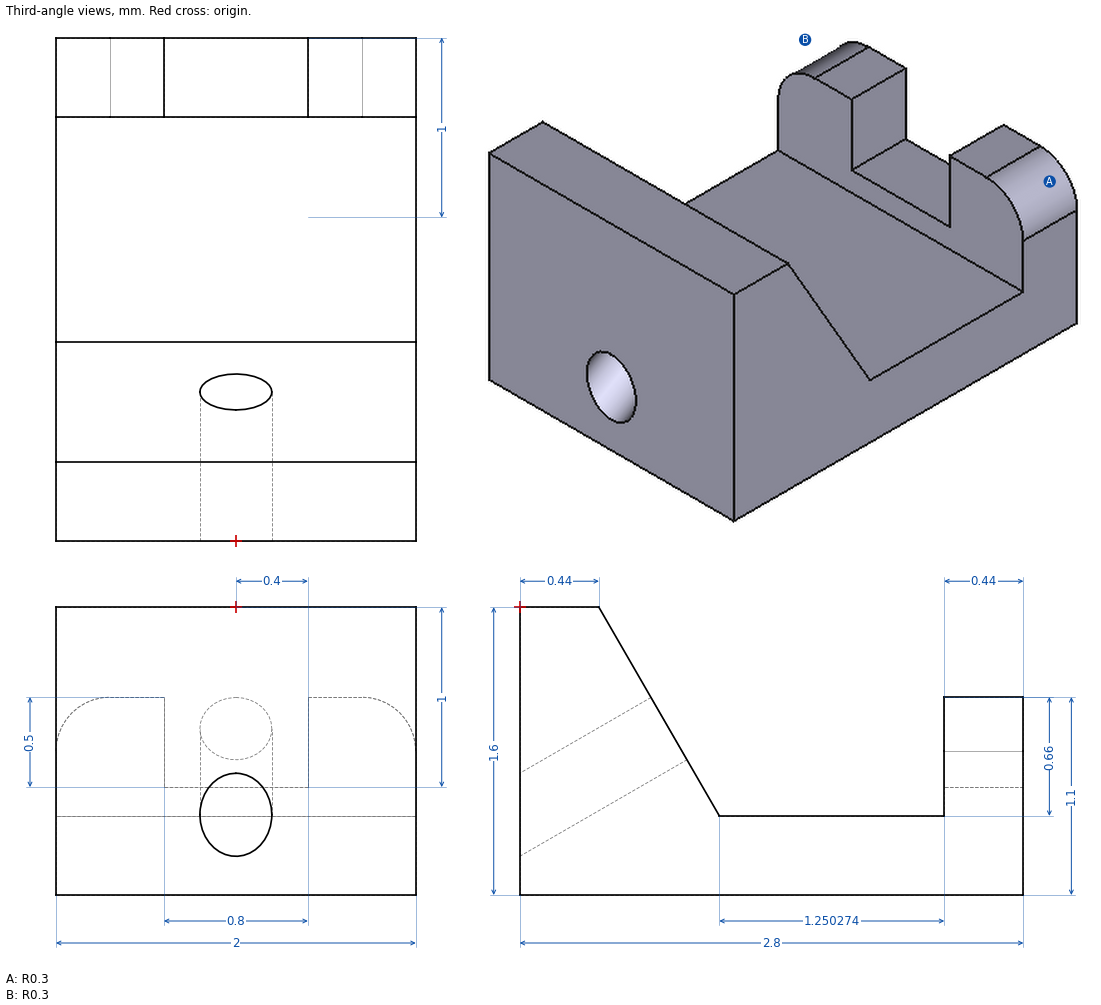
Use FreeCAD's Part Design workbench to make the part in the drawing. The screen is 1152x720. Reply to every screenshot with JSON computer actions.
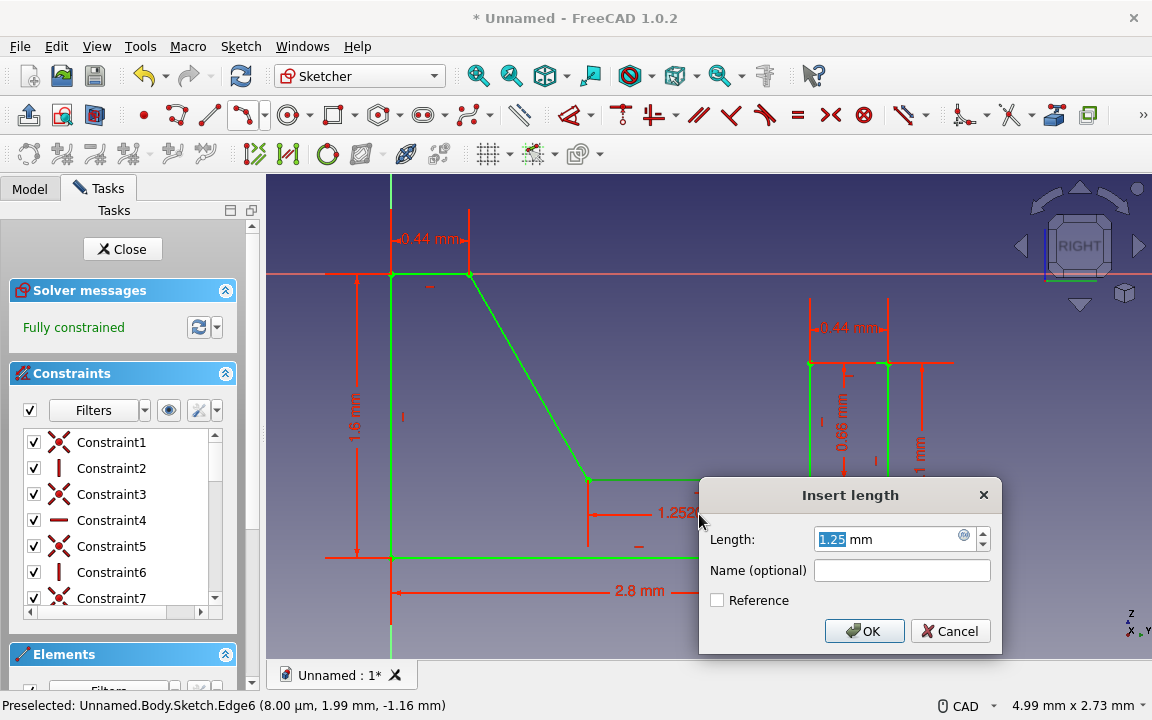
{"action": "type", "text": "1.250274"}
{"action": "key", "text": "Return"}
{"action": "key", "text": "Escape"}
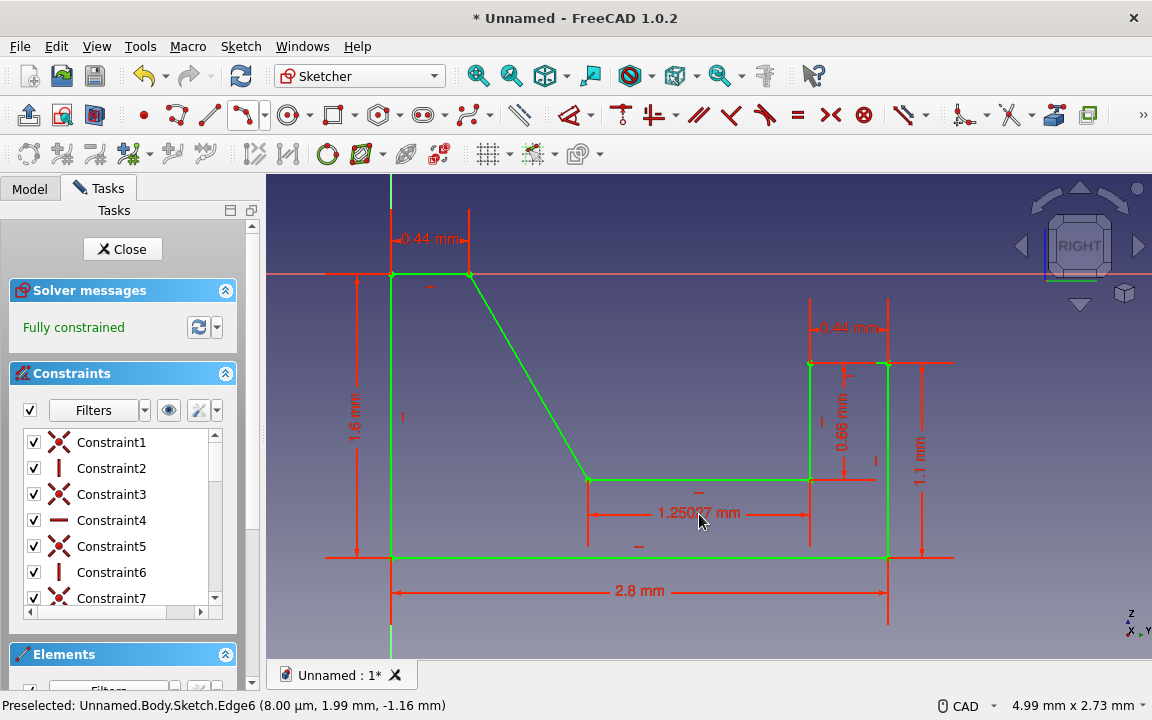
{"action": "left_click", "coordinate": [123, 249]}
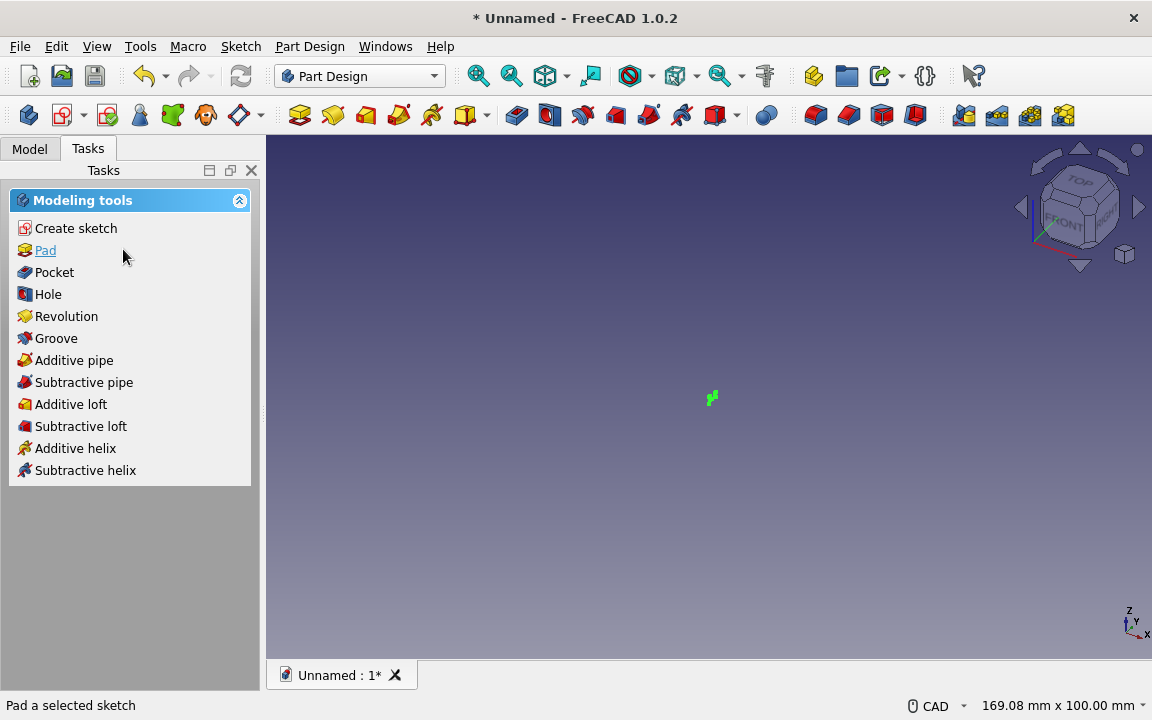
{"action": "left_click", "coordinate": [300, 116]}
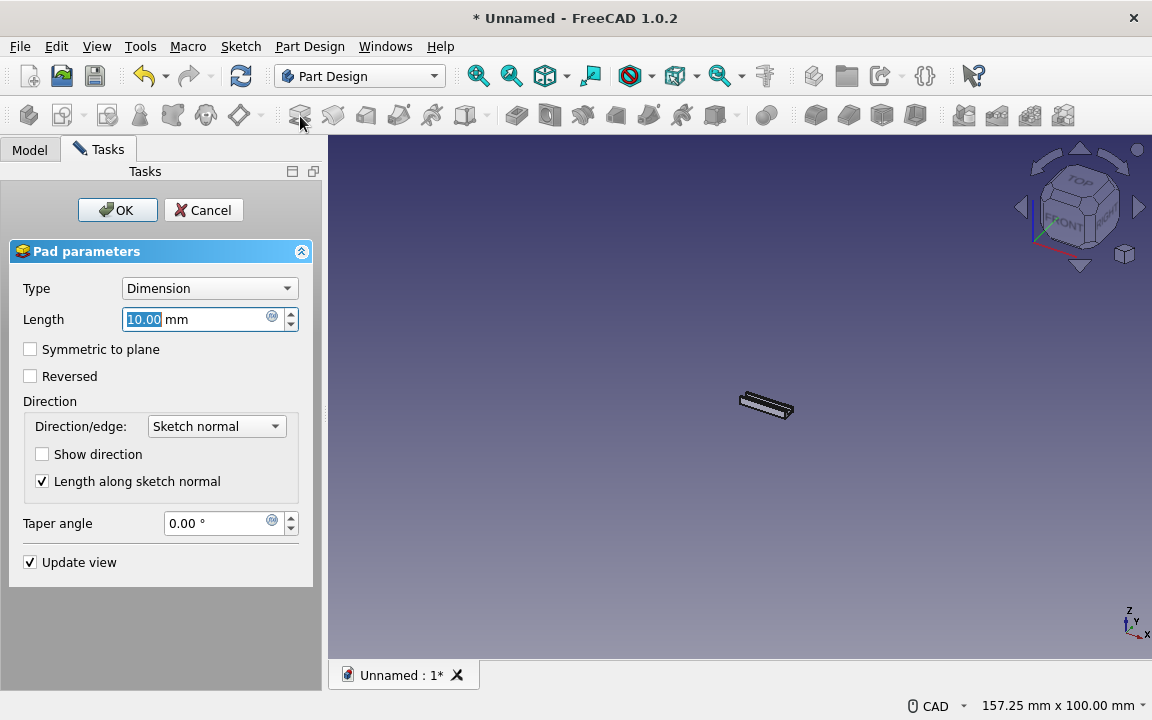
{"action": "type", "text": "2"}
{"action": "key", "text": "Tab"}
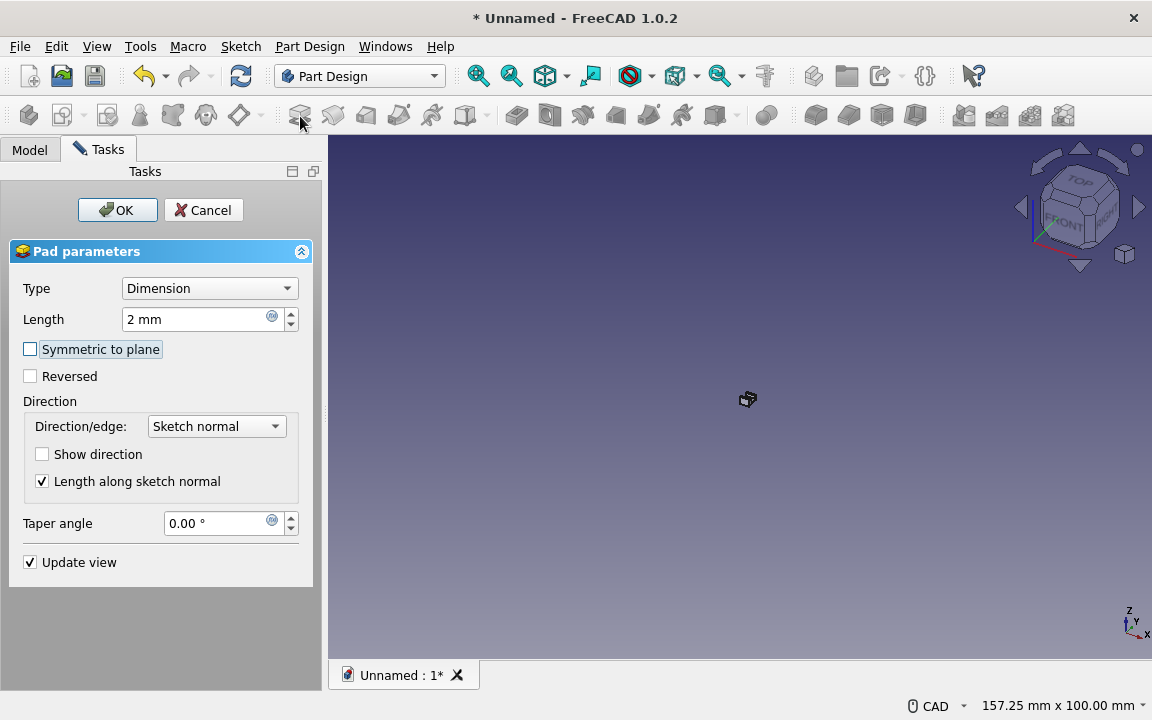
{"action": "left_click", "coordinate": [31, 349]}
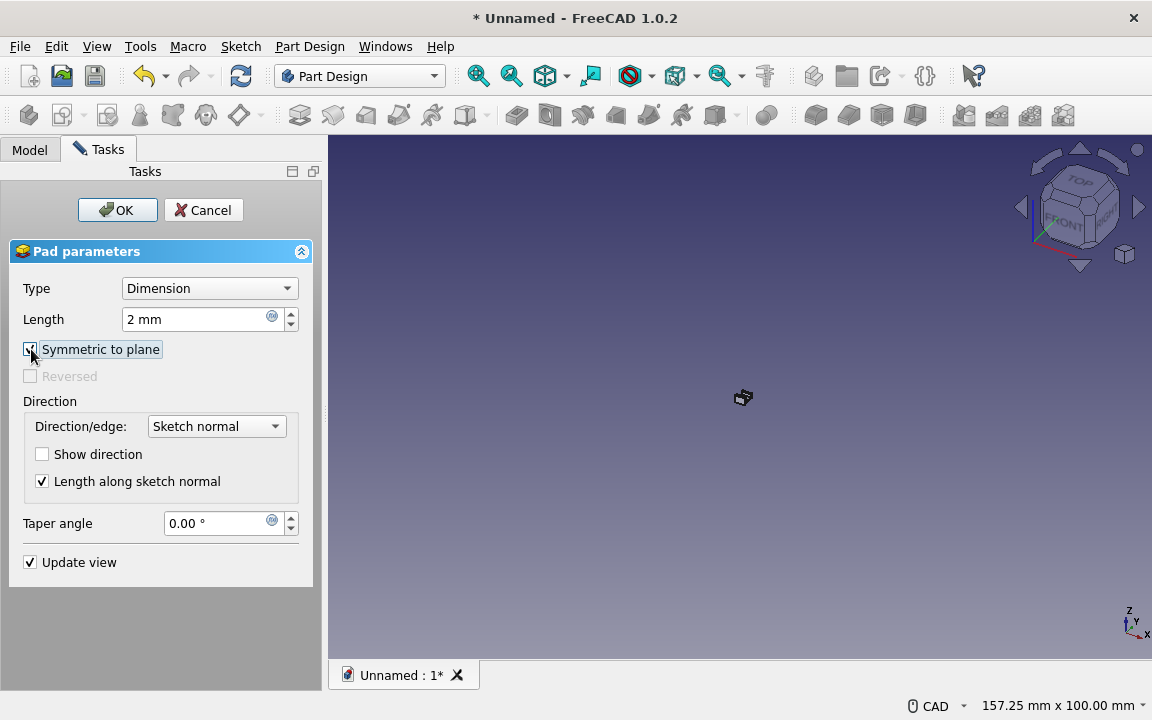
{"action": "left_click", "coordinate": [118, 210]}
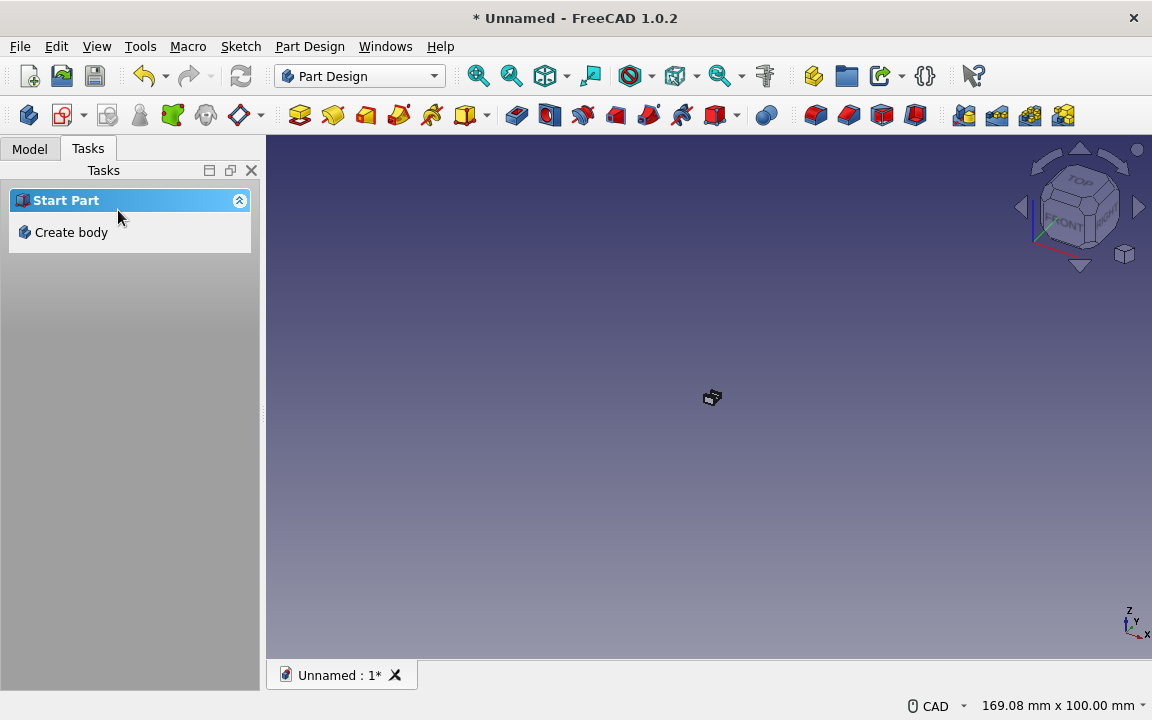
{"action": "key", "text": "v f"}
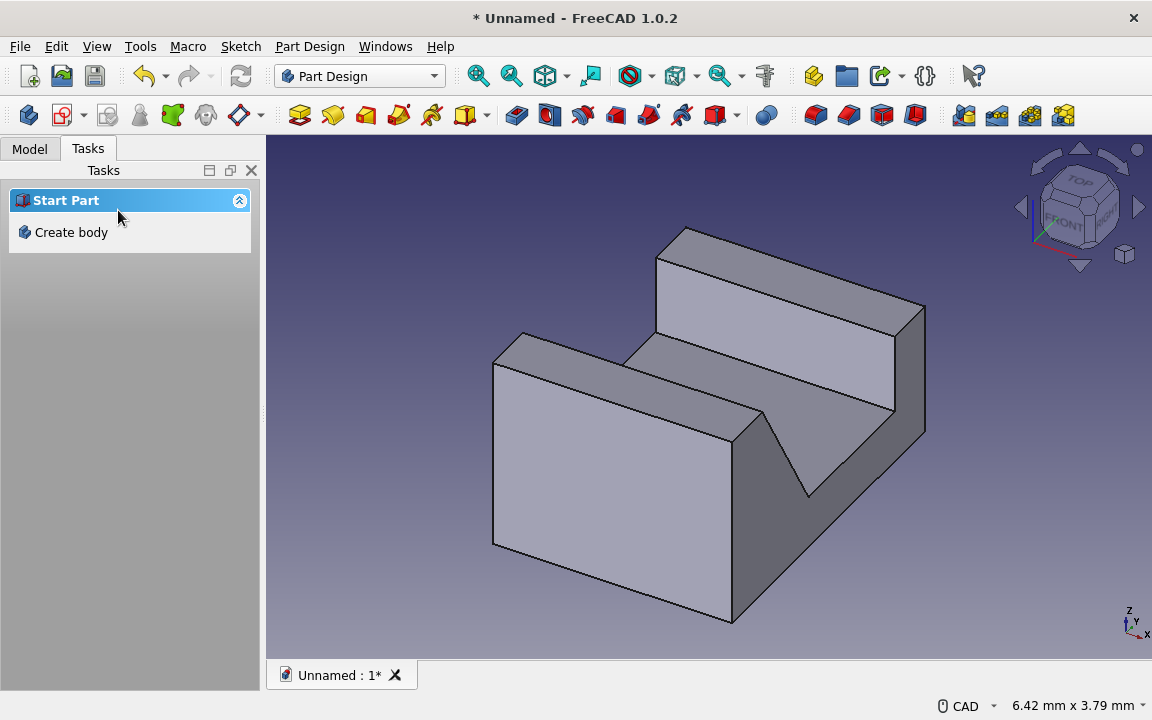
{"action": "key", "text": "4"}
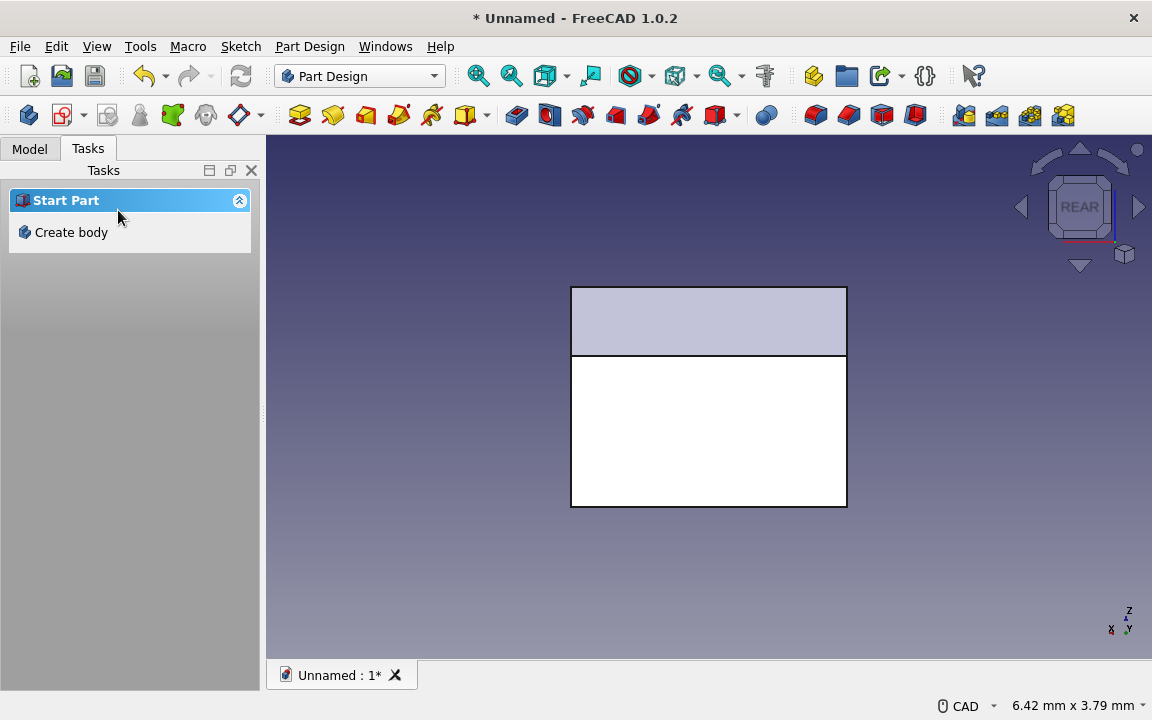
{"action": "key", "text": "v f"}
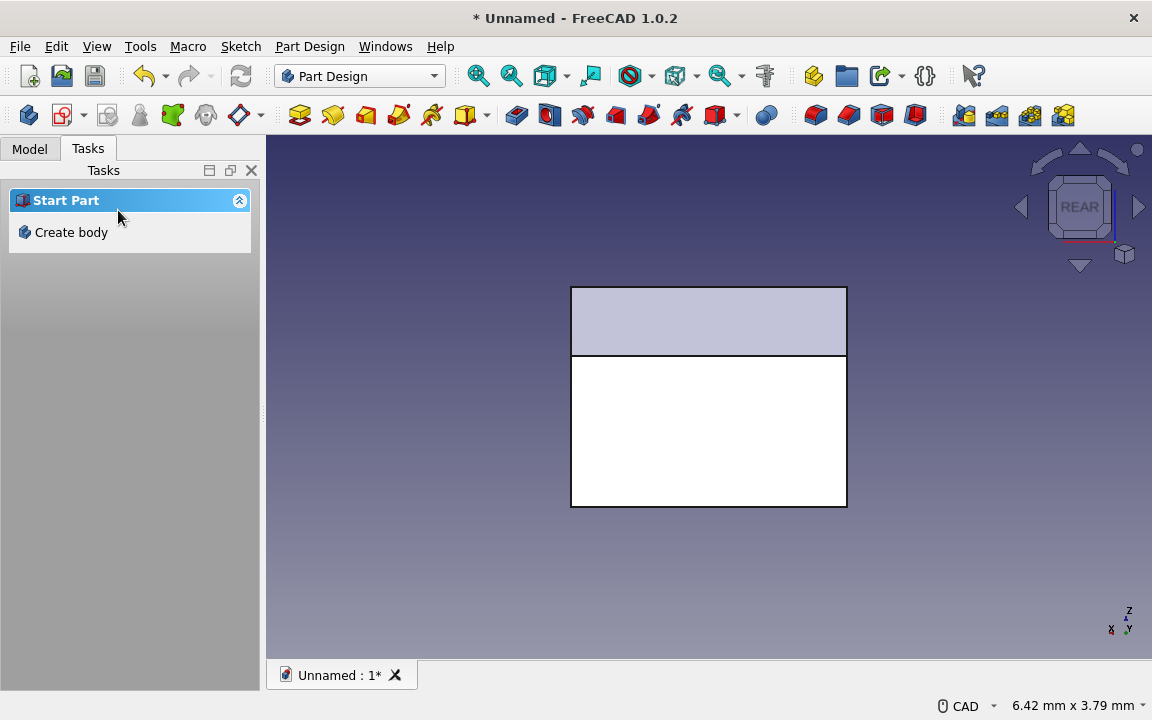
{"action": "left_click", "coordinate": [709, 431]}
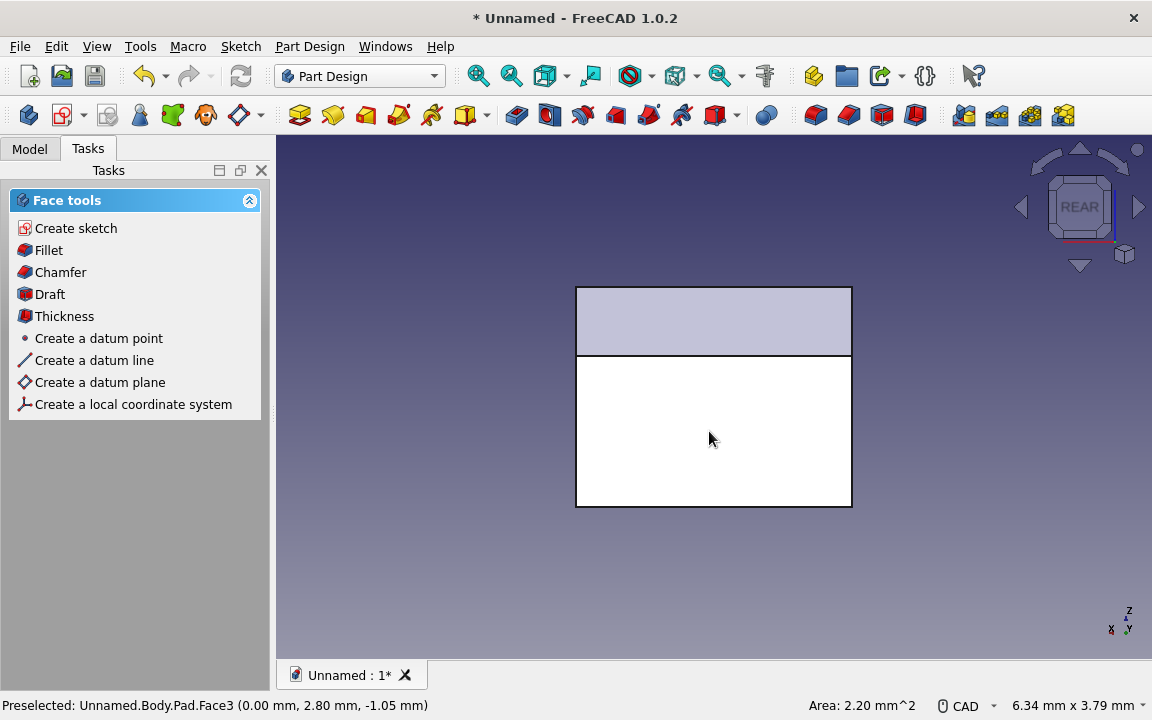
{"action": "left_click", "coordinate": [62, 116]}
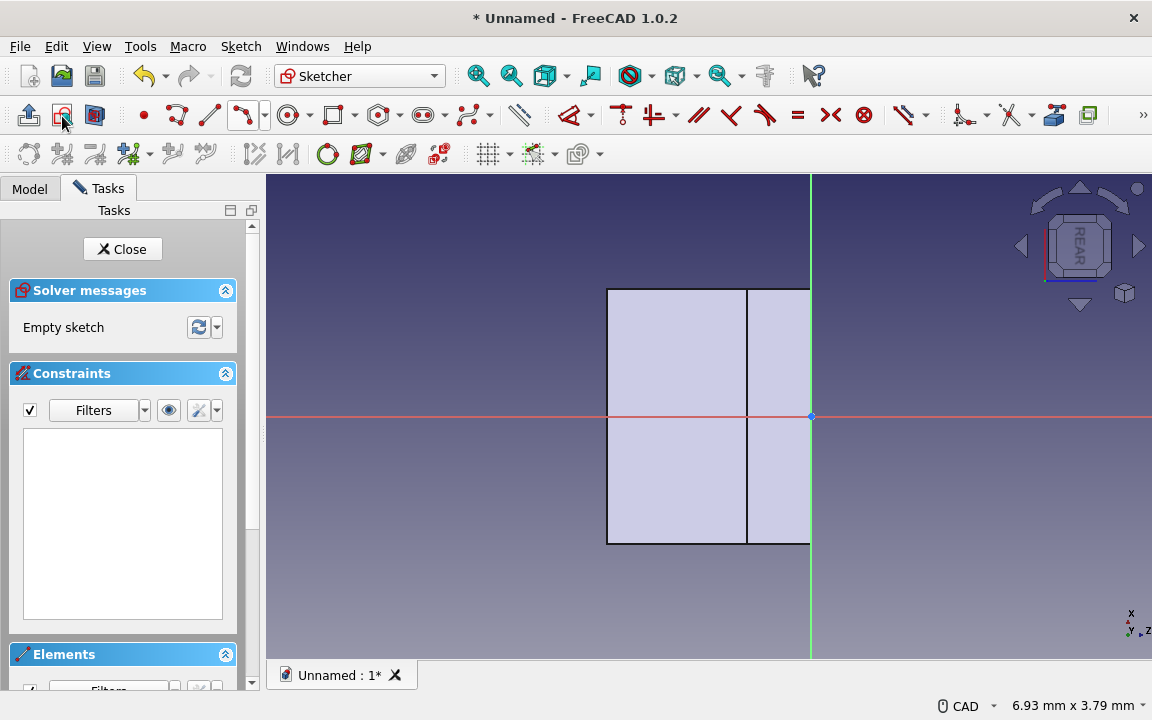
{"action": "scroll", "coordinate": [810, 416], "scroll_direction": "up", "scroll_amount": 5}